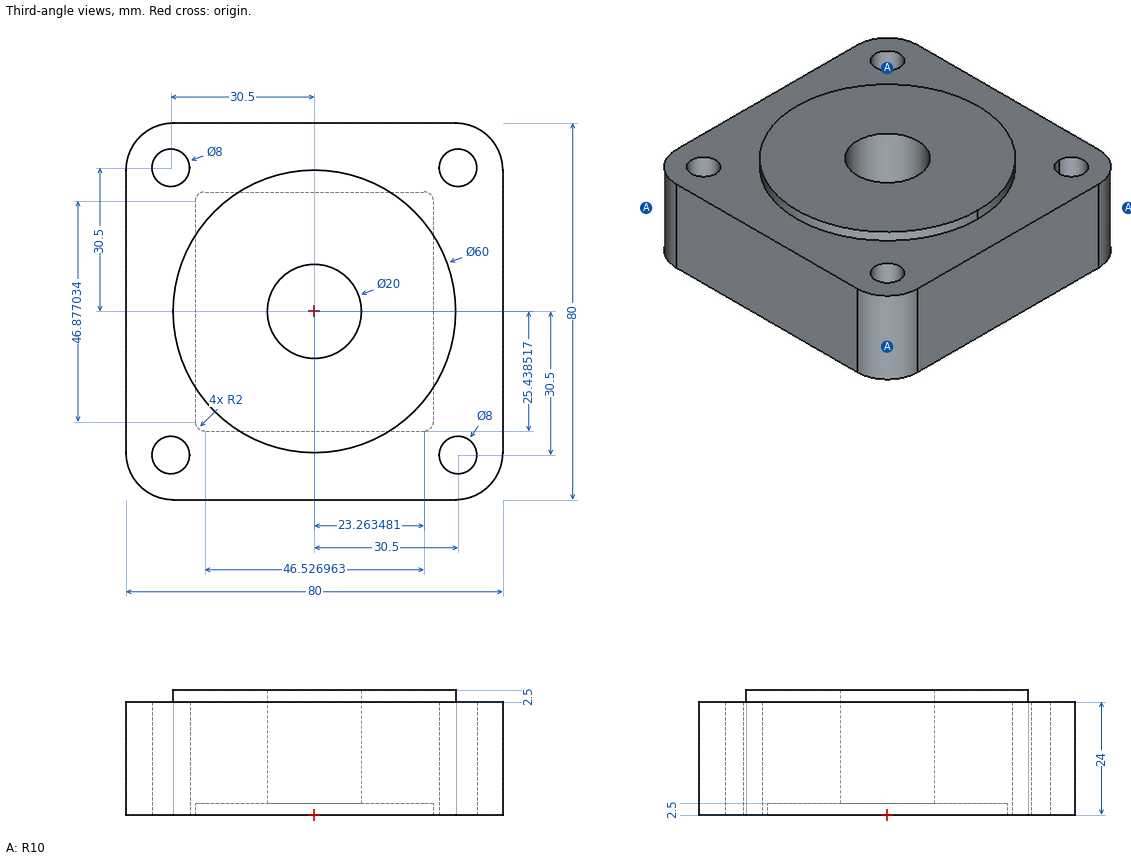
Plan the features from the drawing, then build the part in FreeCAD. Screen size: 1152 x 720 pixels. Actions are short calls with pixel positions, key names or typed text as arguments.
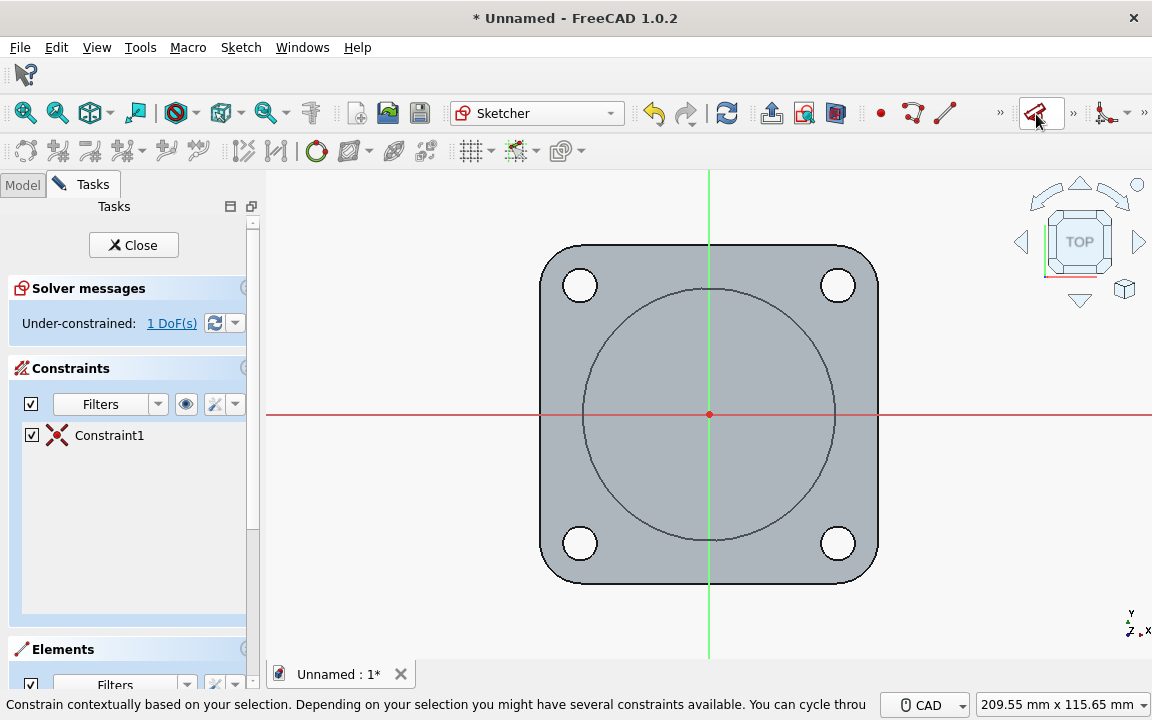
click(798, 325)
click(821, 302)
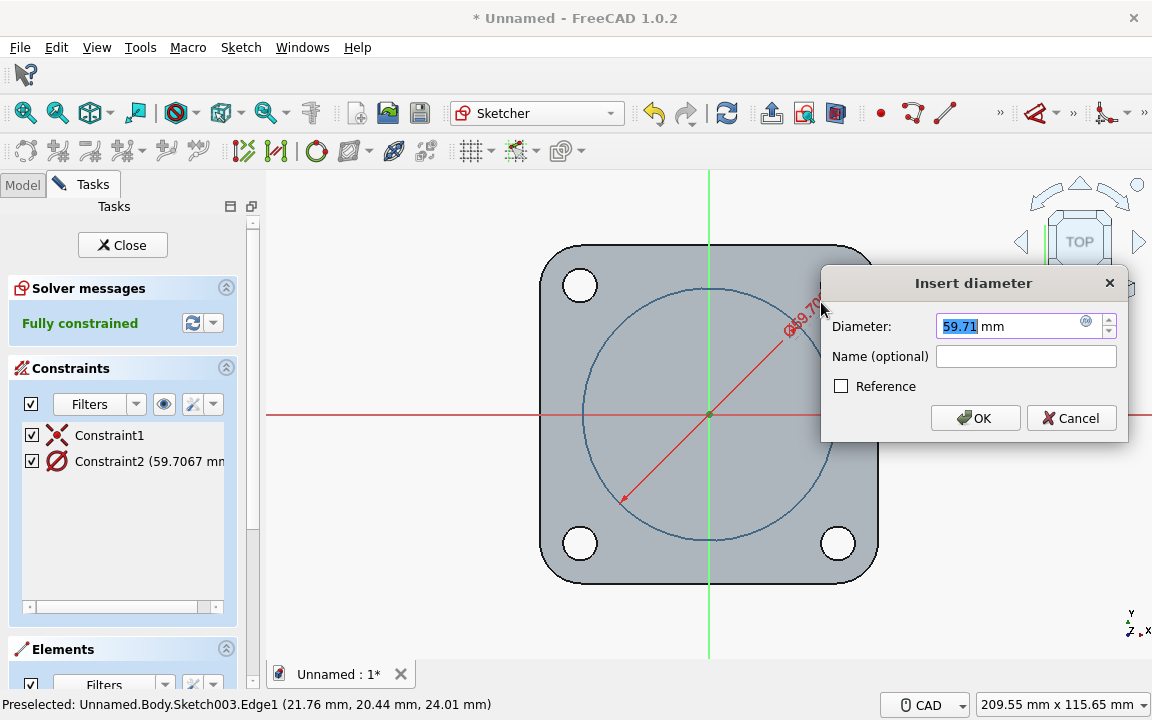
text(60)
key(Return)
key(Escape)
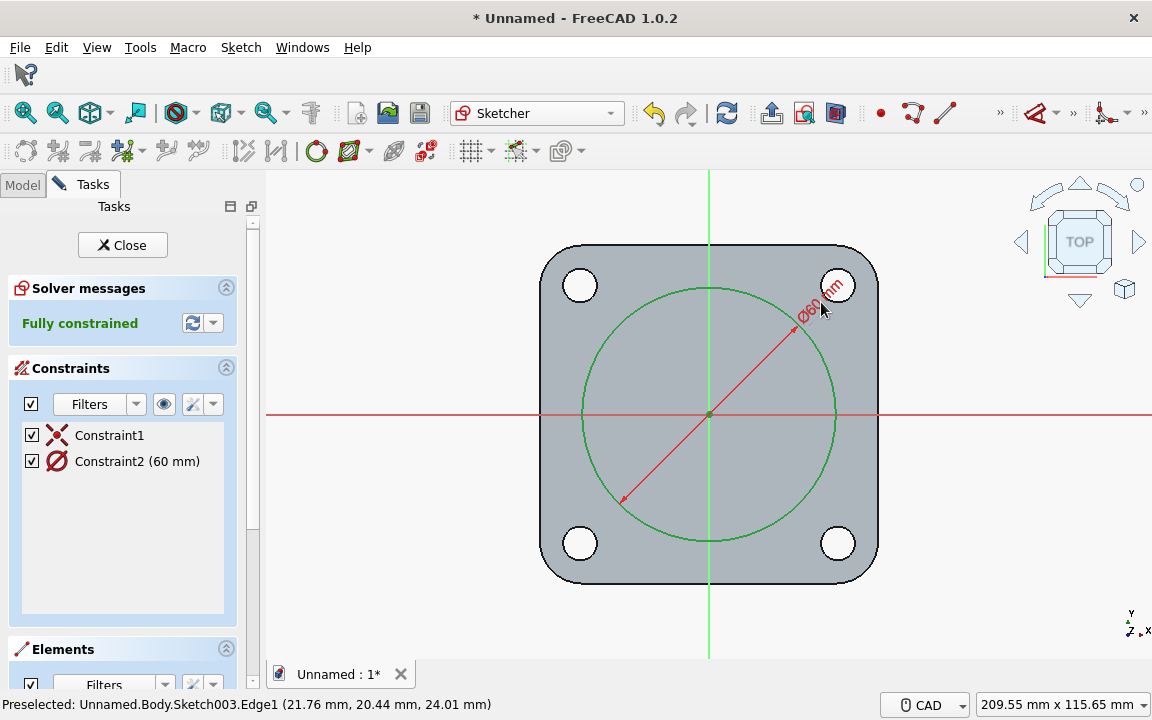
click(123, 245)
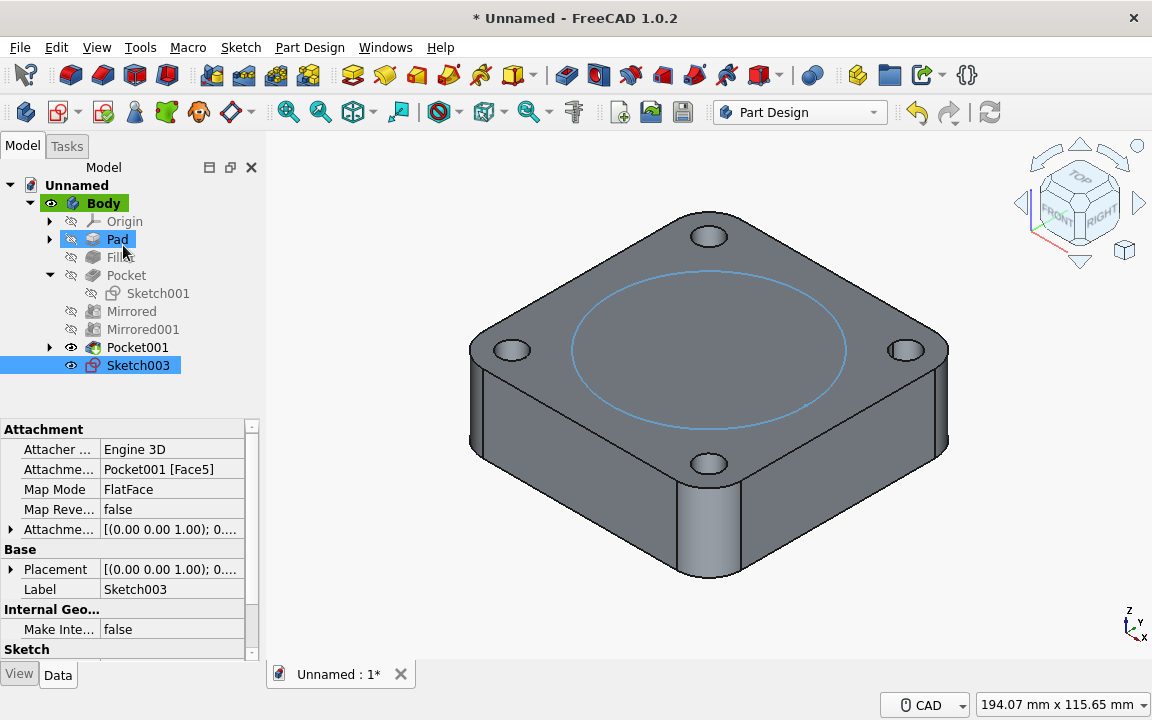
click(354, 76)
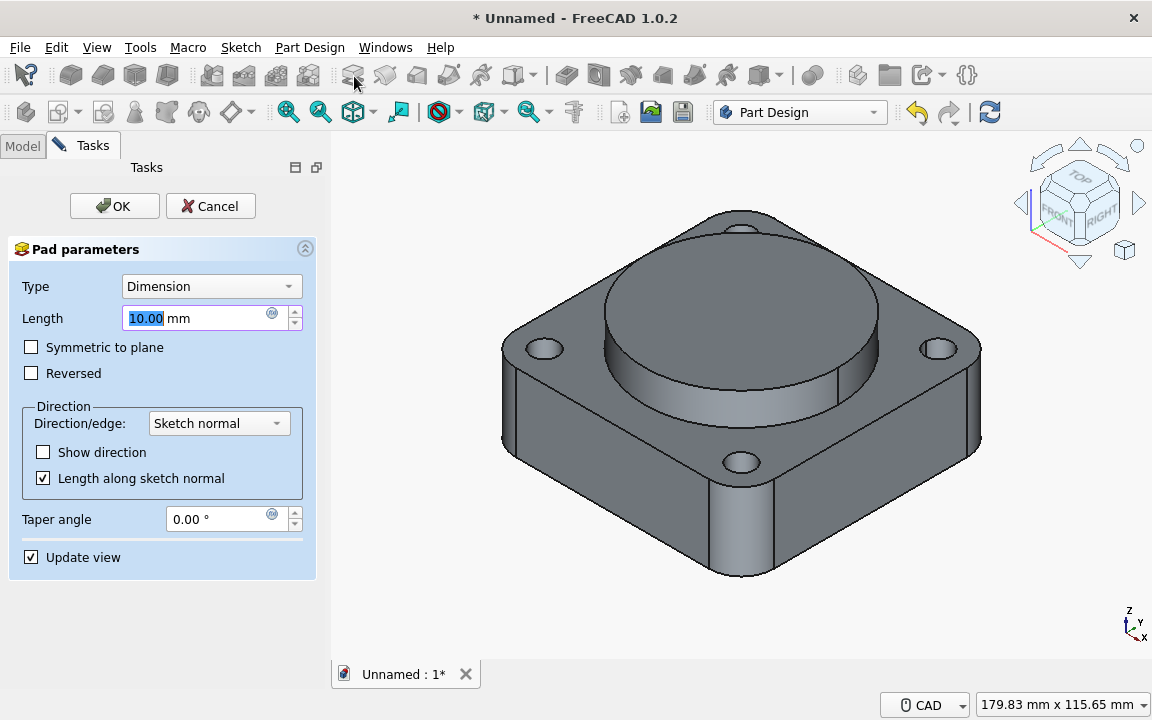
text(2.5)
key(Tab)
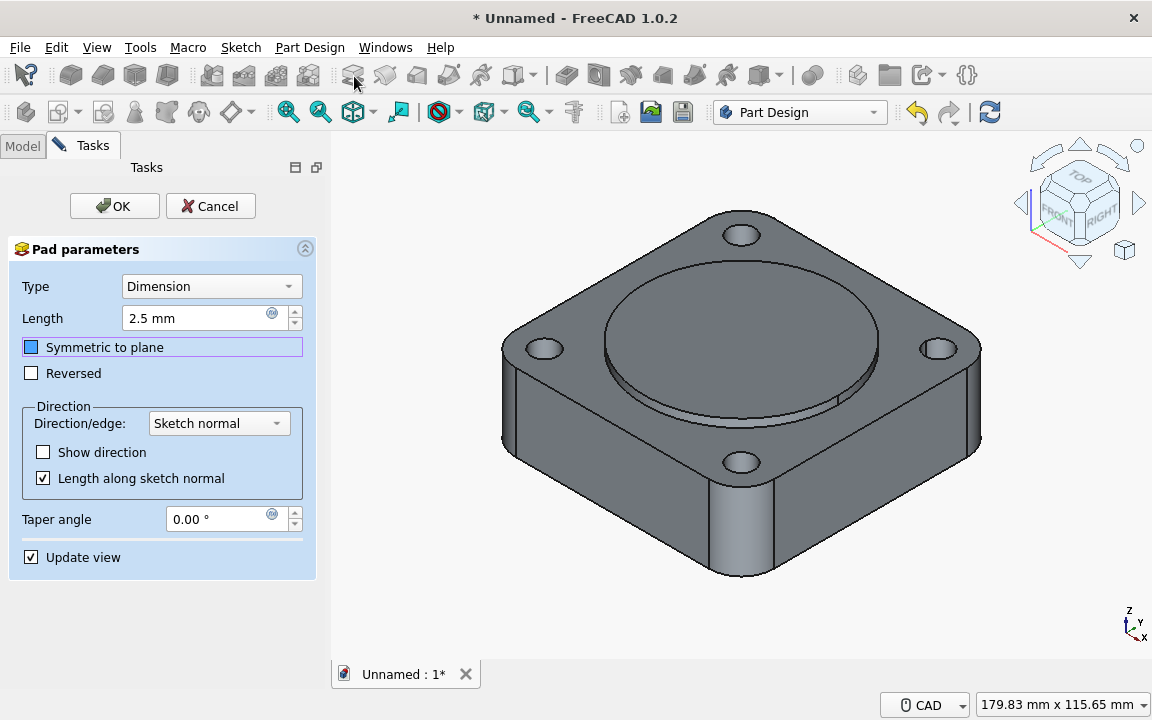
click(115, 206)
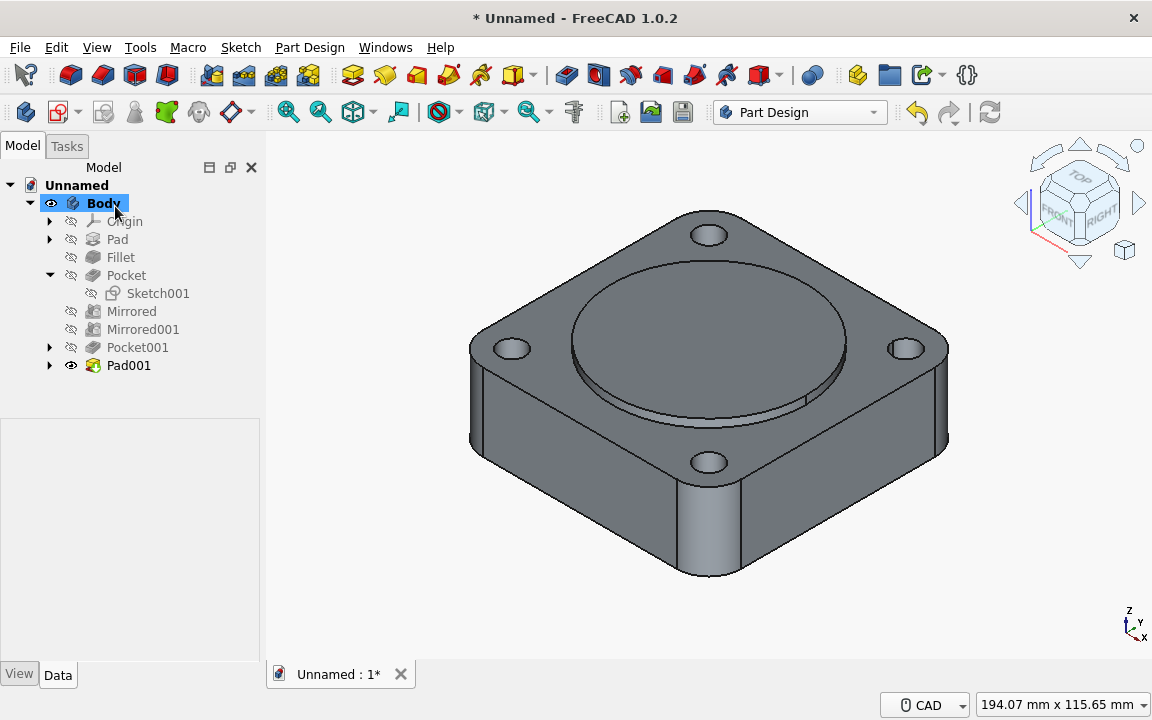
click(709, 339)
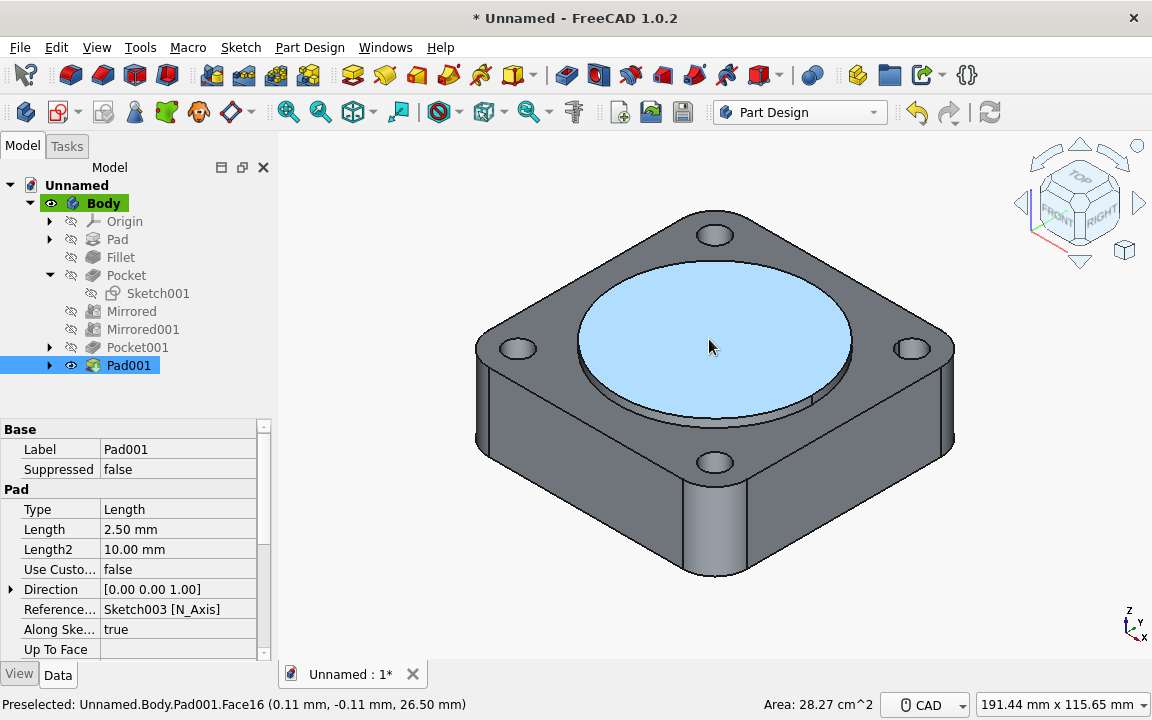
click(58, 112)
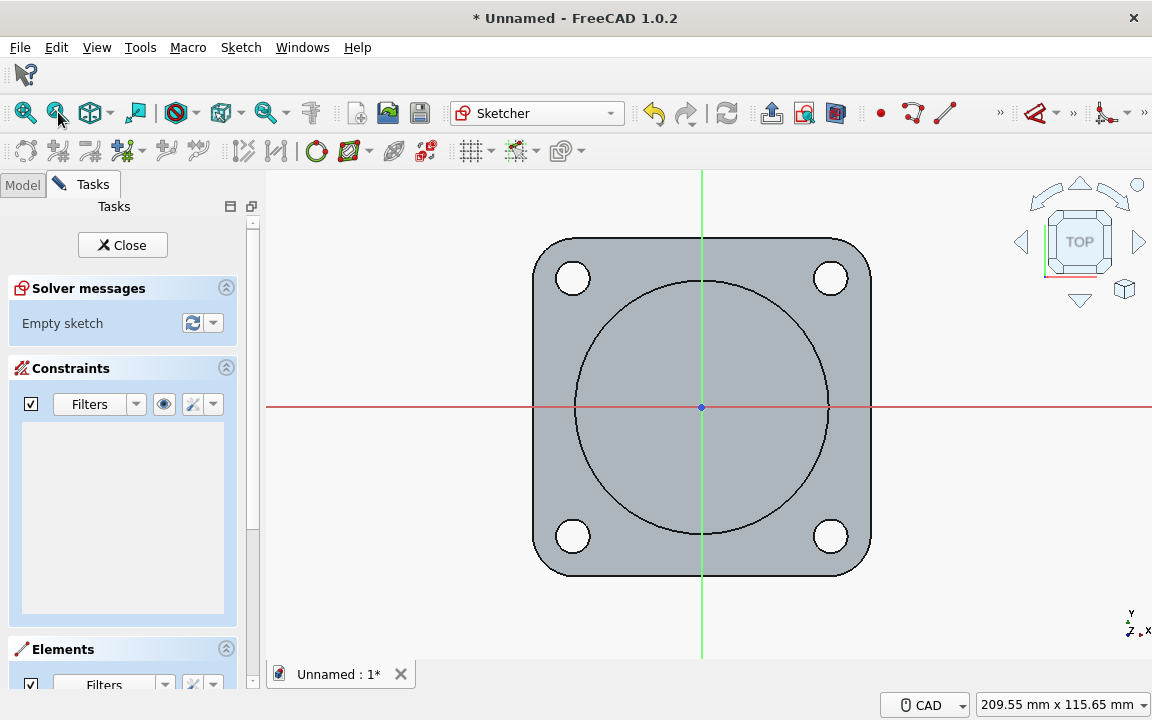
scroll(728, 404, up, 6)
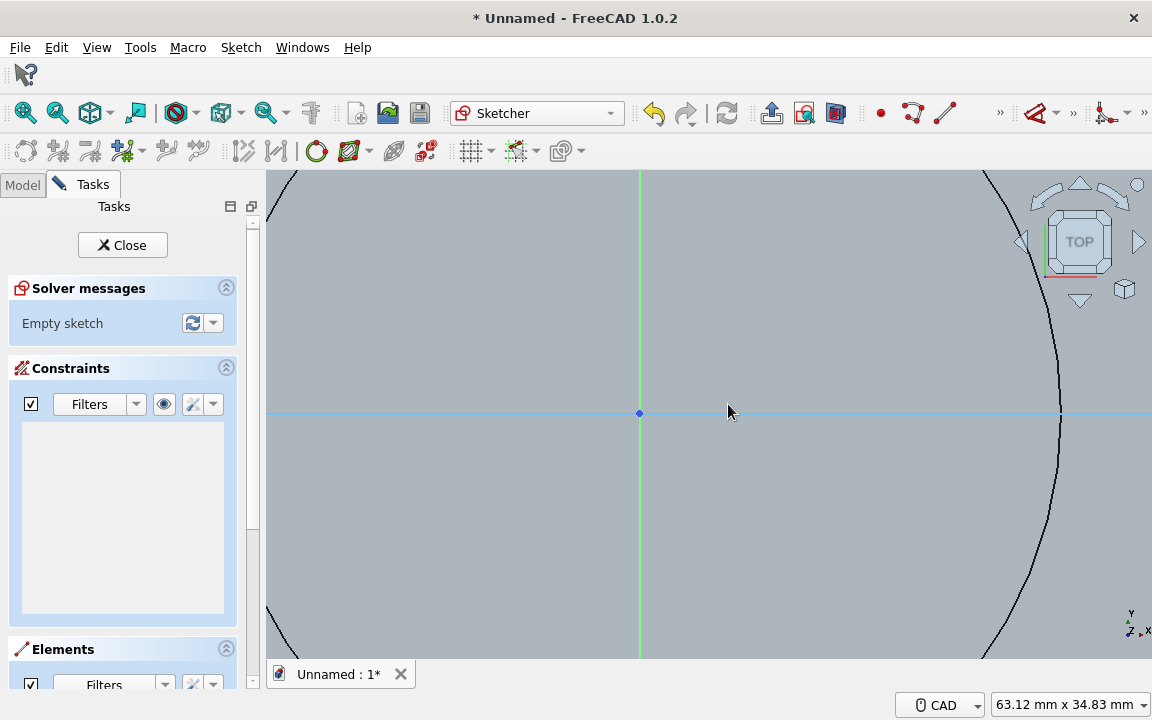
key(g)
key(c)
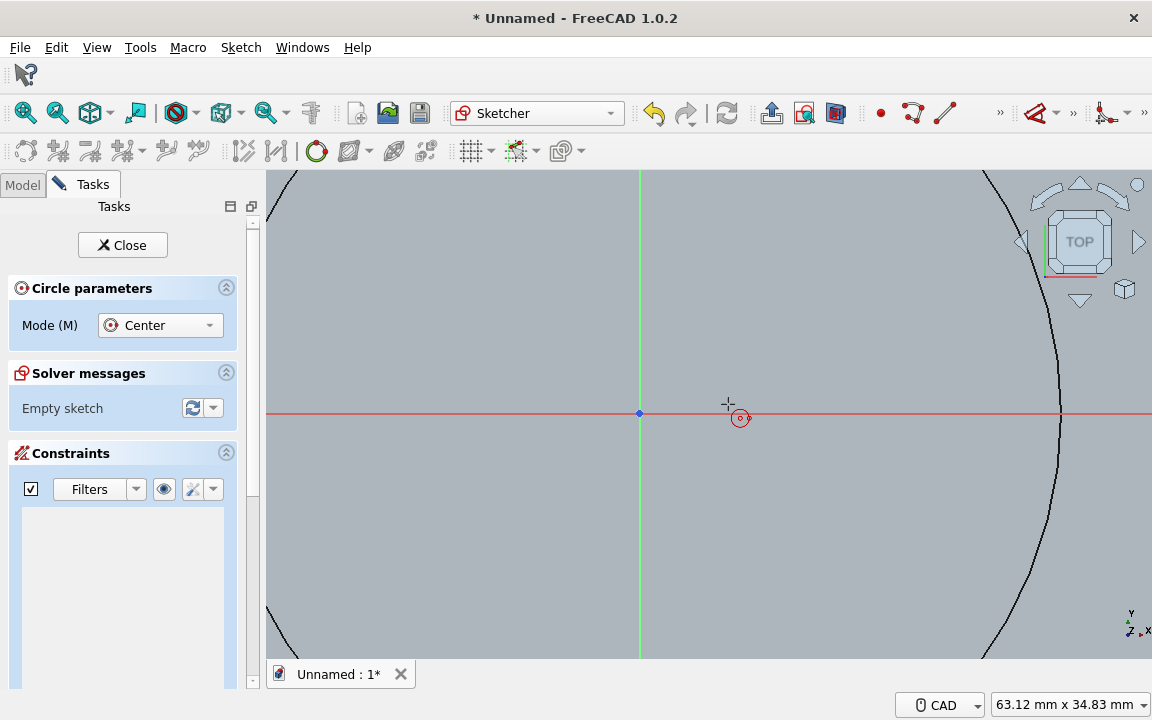
click(640, 414)
click(739, 315)
key(Escape)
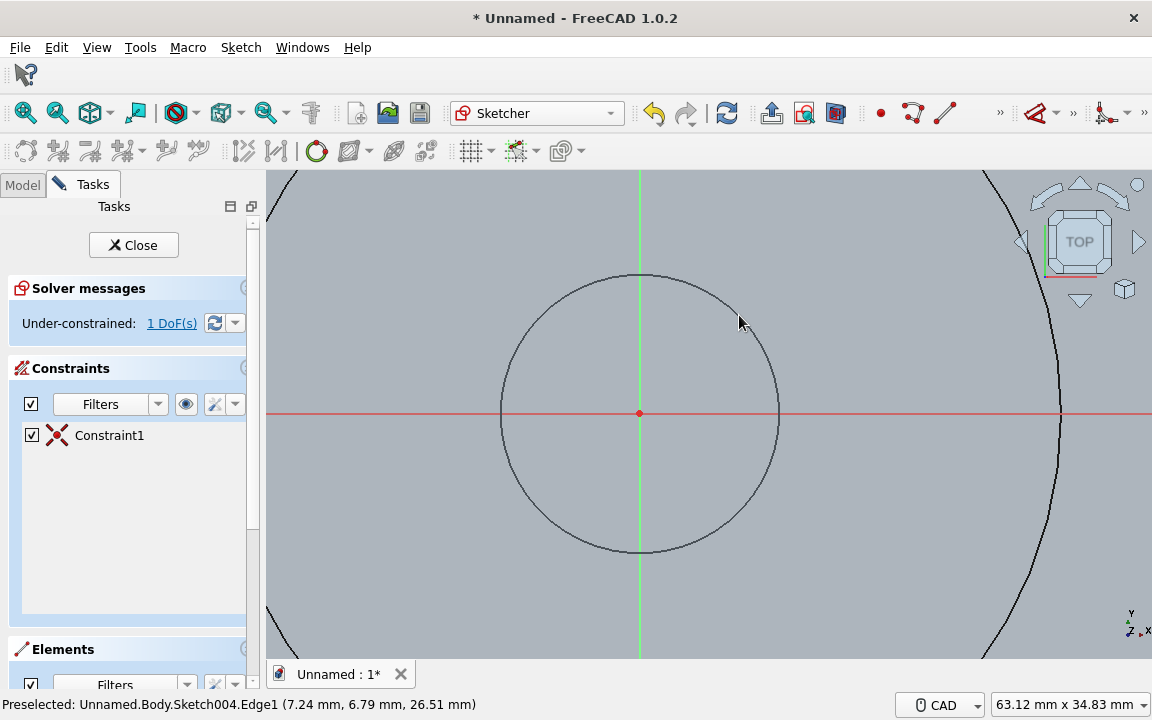
click(1036, 114)